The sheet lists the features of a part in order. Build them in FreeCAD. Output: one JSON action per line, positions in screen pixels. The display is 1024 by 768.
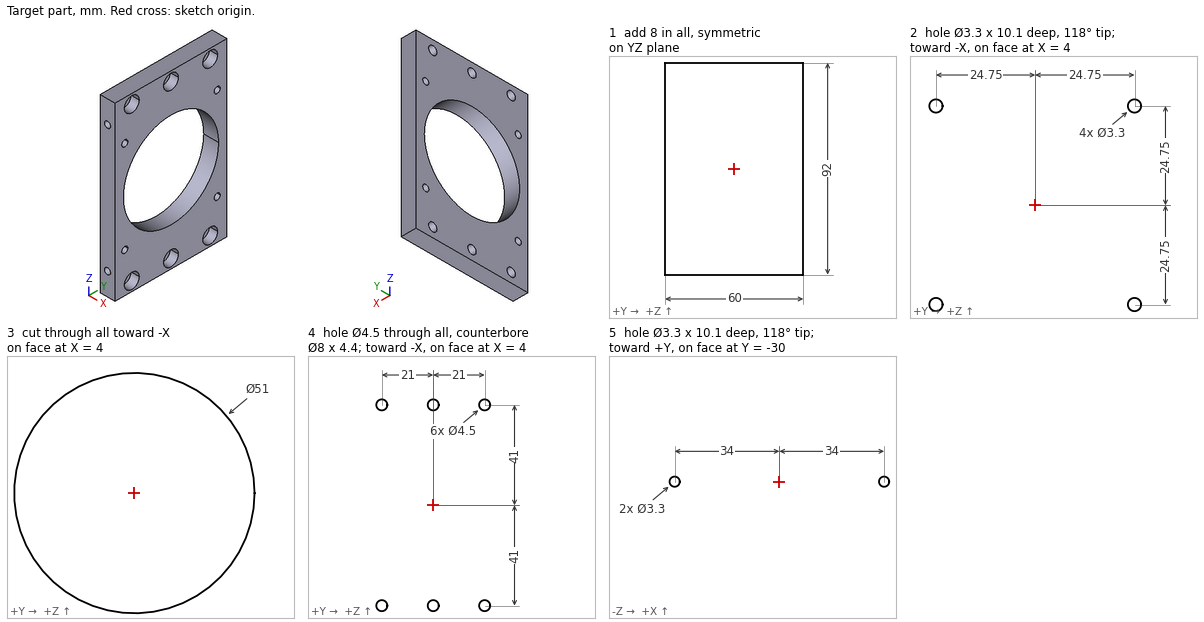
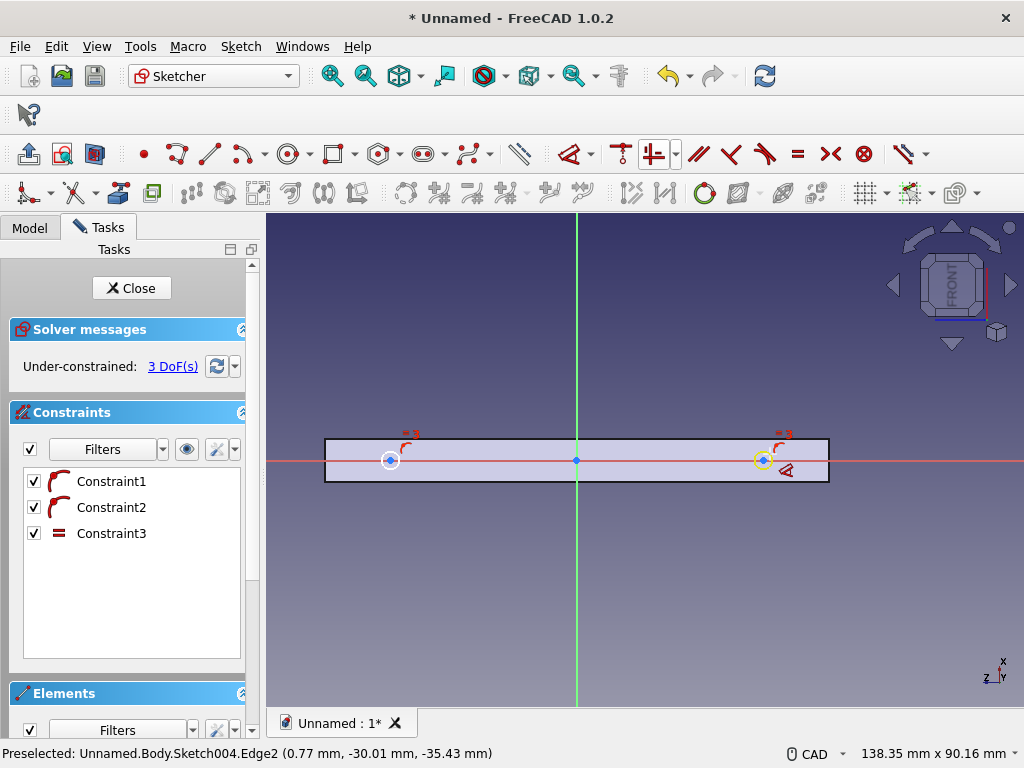
{"action": "scroll", "coordinate": [397, 454], "scroll_direction": "up", "scroll_amount": 4}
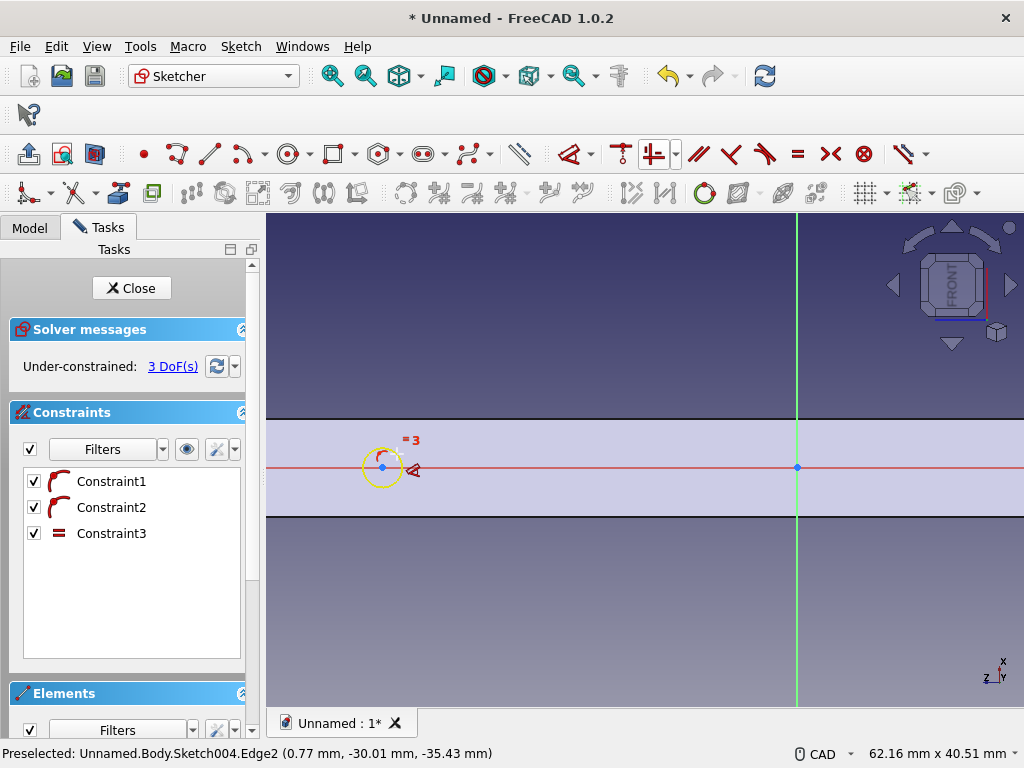
{"action": "left_click", "coordinate": [396, 454]}
{"action": "left_click", "coordinate": [418, 431]}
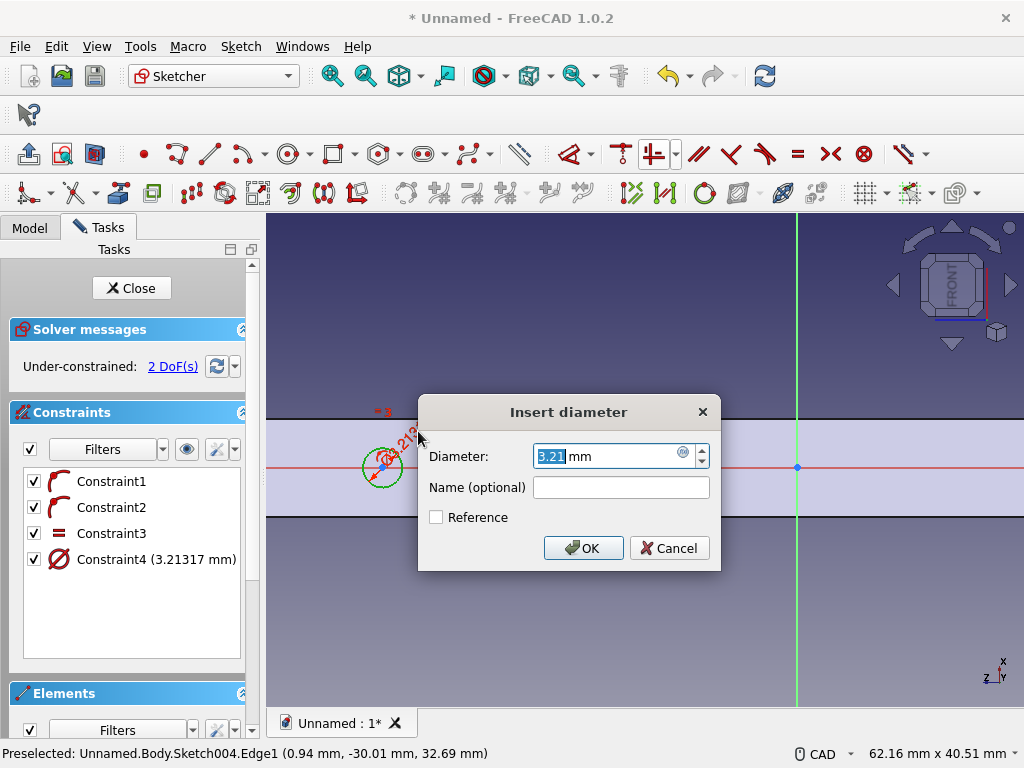
{"action": "type", "text": "3.3"}
{"action": "key", "text": "Return"}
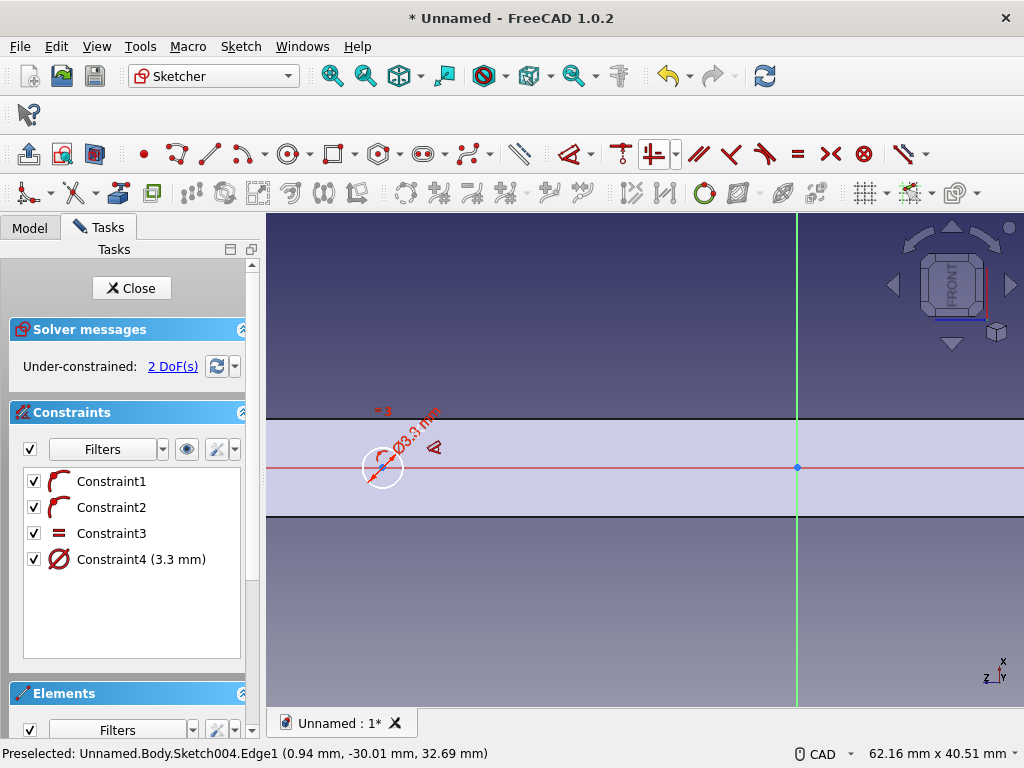
{"action": "left_click", "coordinate": [383, 468]}
{"action": "left_click", "coordinate": [590, 502]}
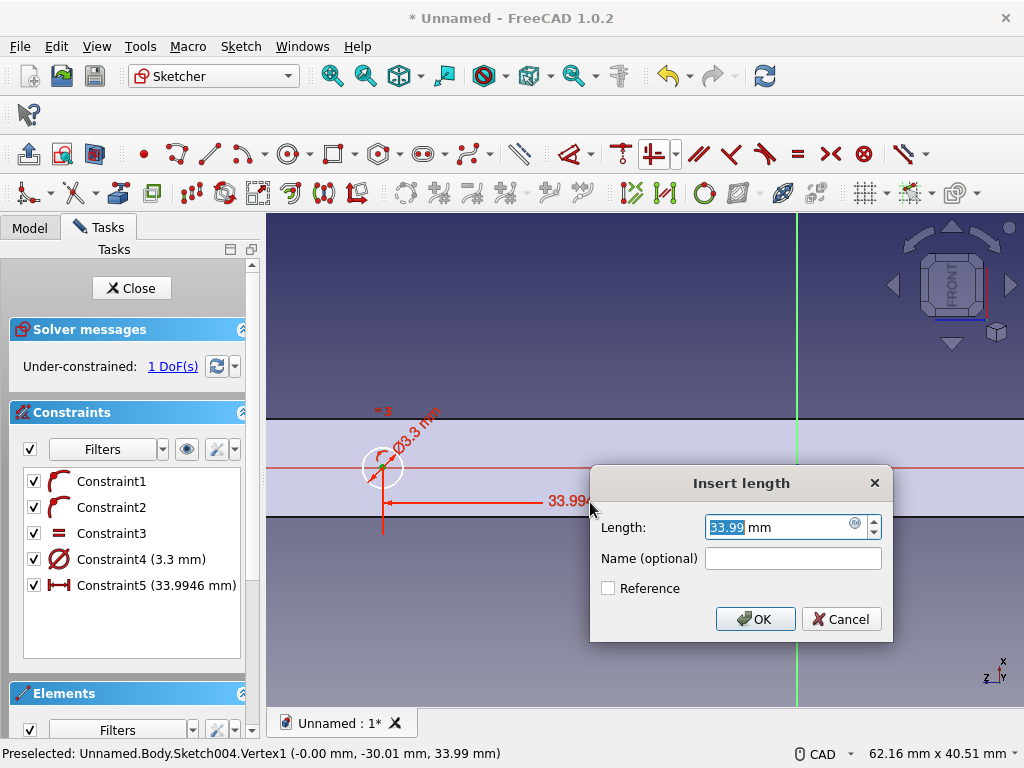
{"action": "type", "text": "34"}
{"action": "key", "text": "Return"}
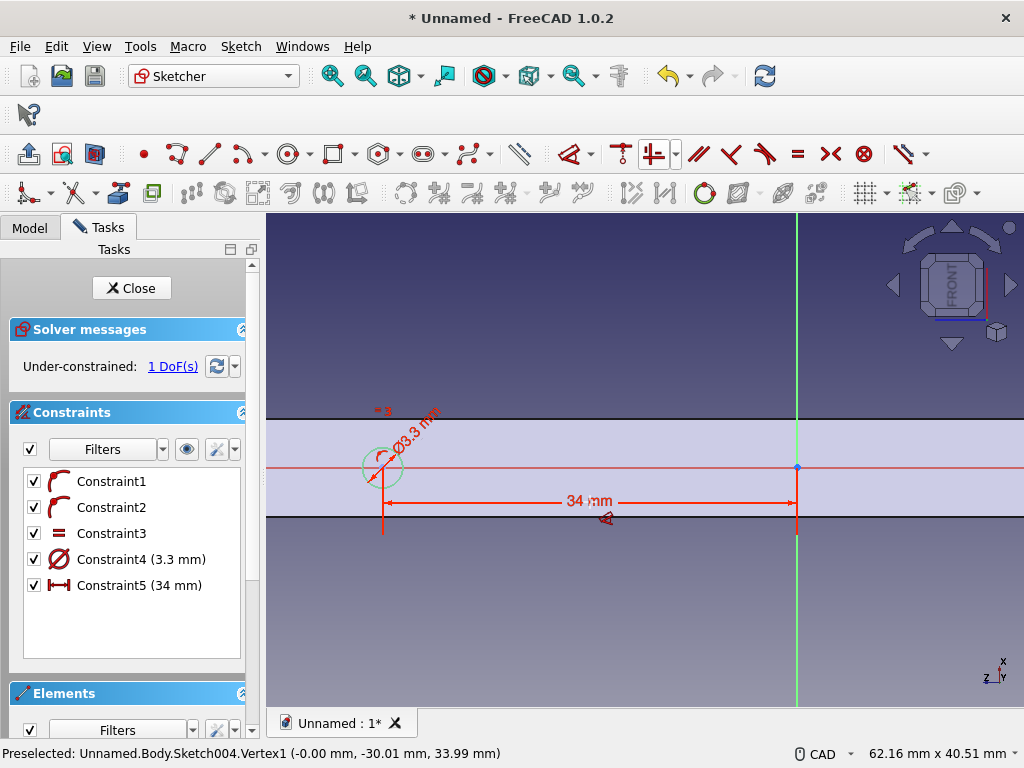
{"action": "scroll", "coordinate": [396, 454], "scroll_direction": "down", "scroll_amount": 4}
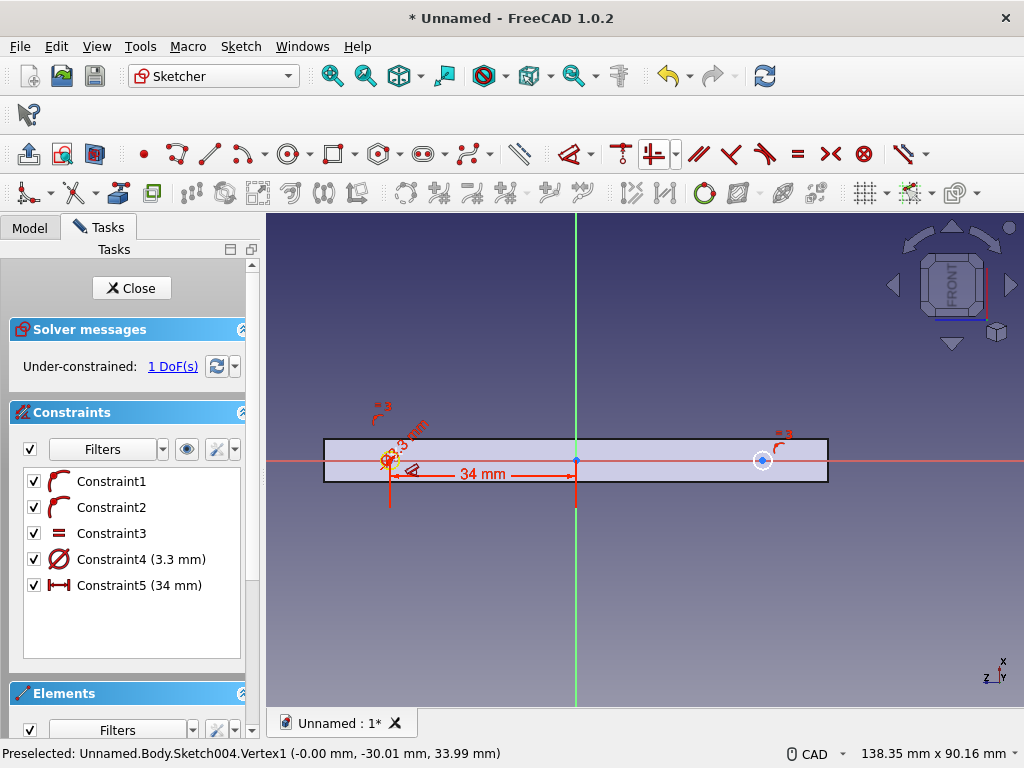
{"action": "left_click", "coordinate": [763, 461]}
{"action": "left_click", "coordinate": [670, 495]}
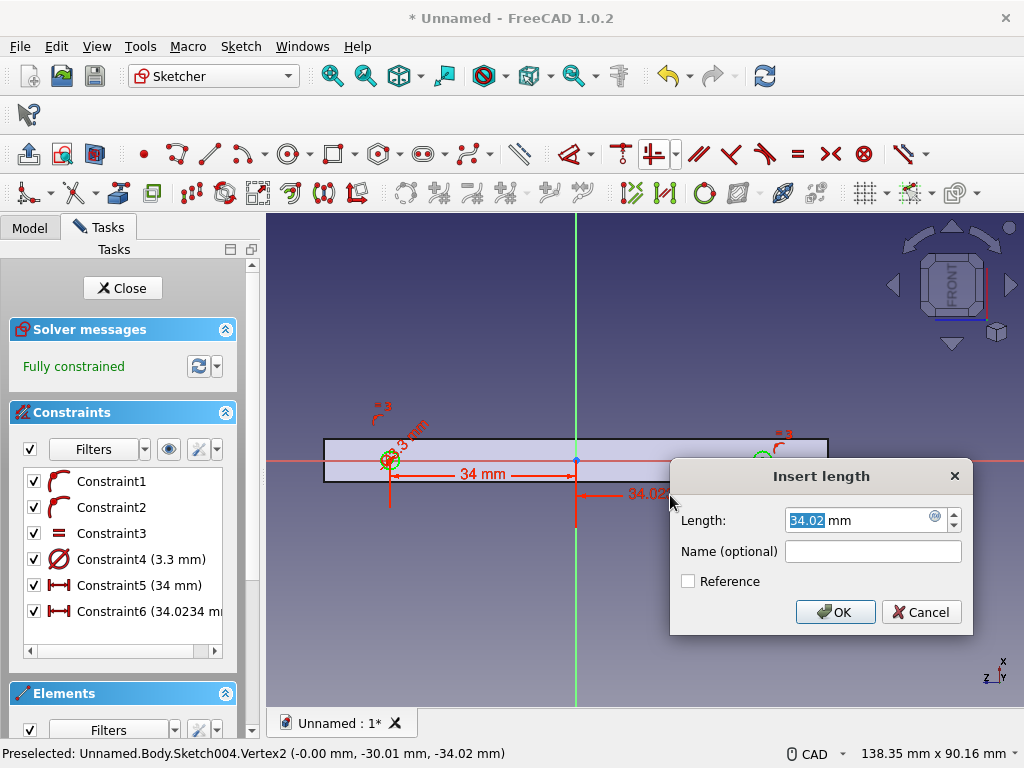
{"action": "type", "text": "34"}
{"action": "key", "text": "Return"}
{"action": "key", "text": "Escape"}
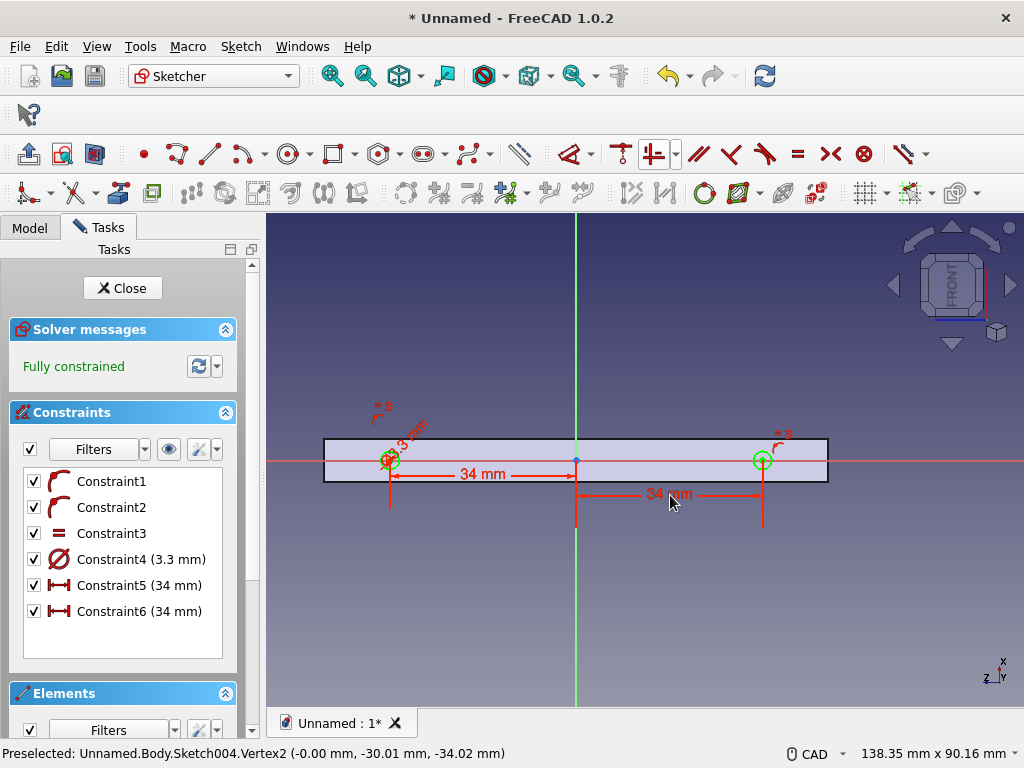
{"action": "left_click", "coordinate": [123, 288]}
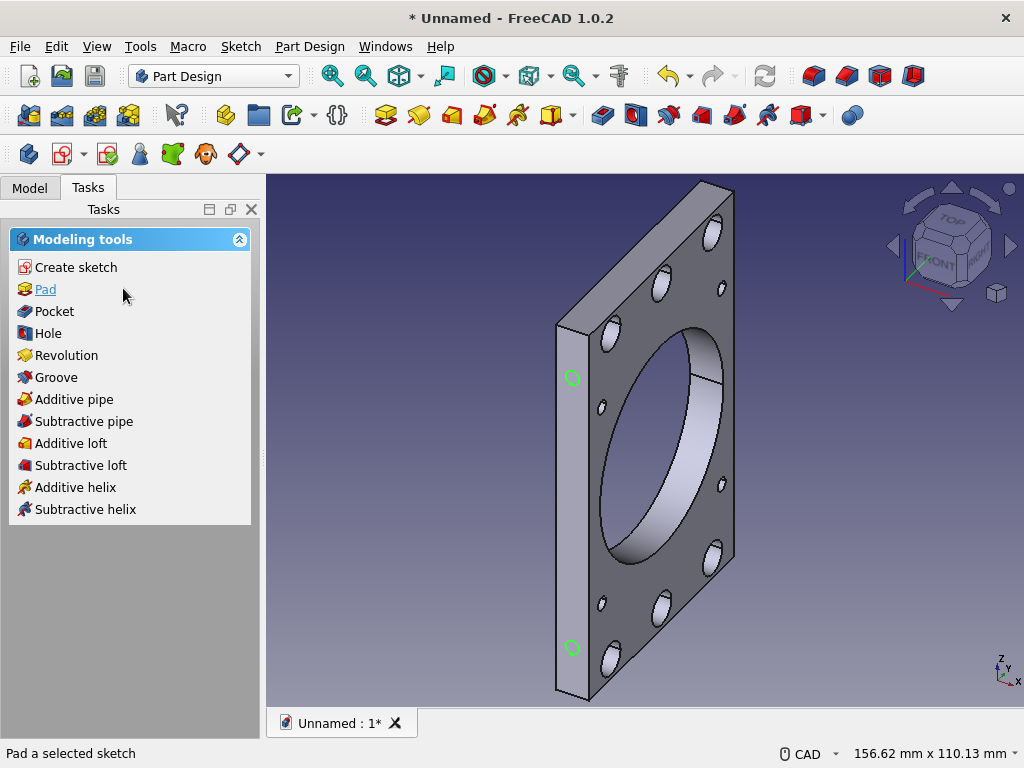
{"action": "left_click", "coordinate": [636, 116]}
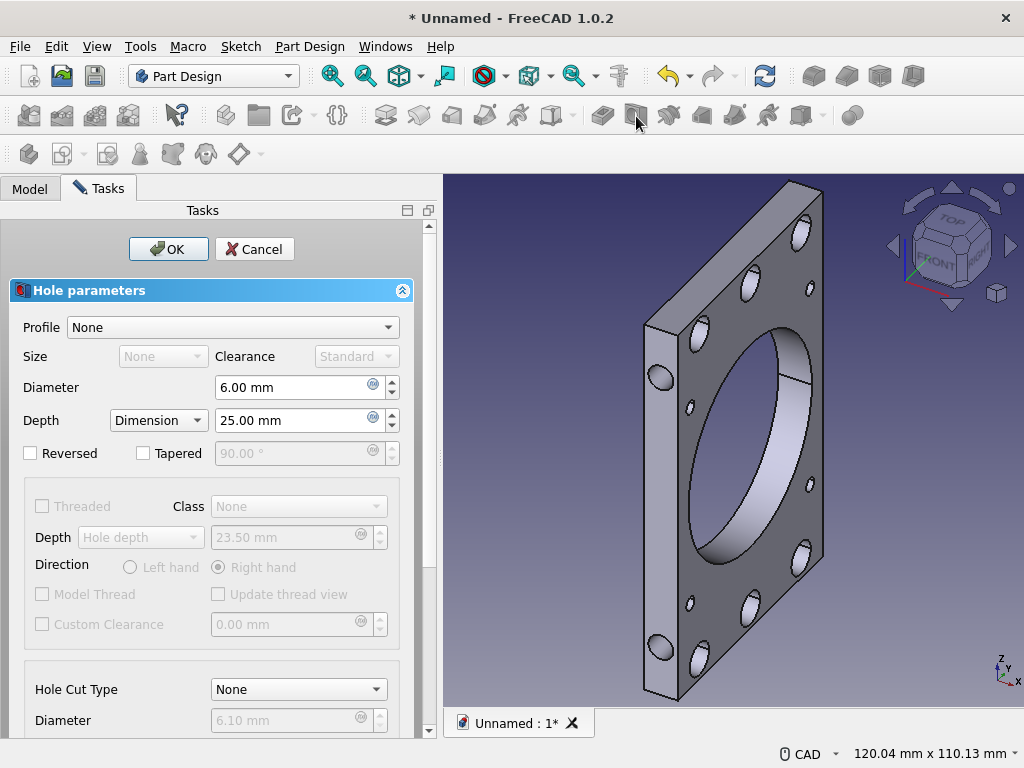
{"action": "triple_click", "coordinate": [300, 388]}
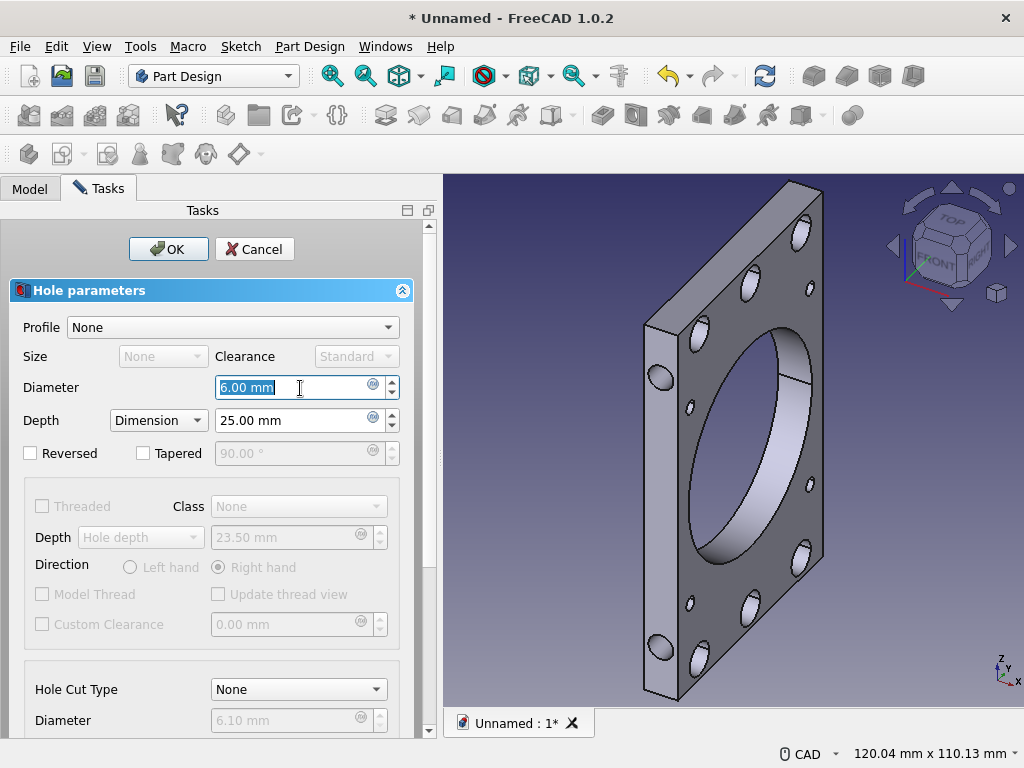
{"action": "type", "text": "3.3"}
{"action": "key", "text": "Tab"}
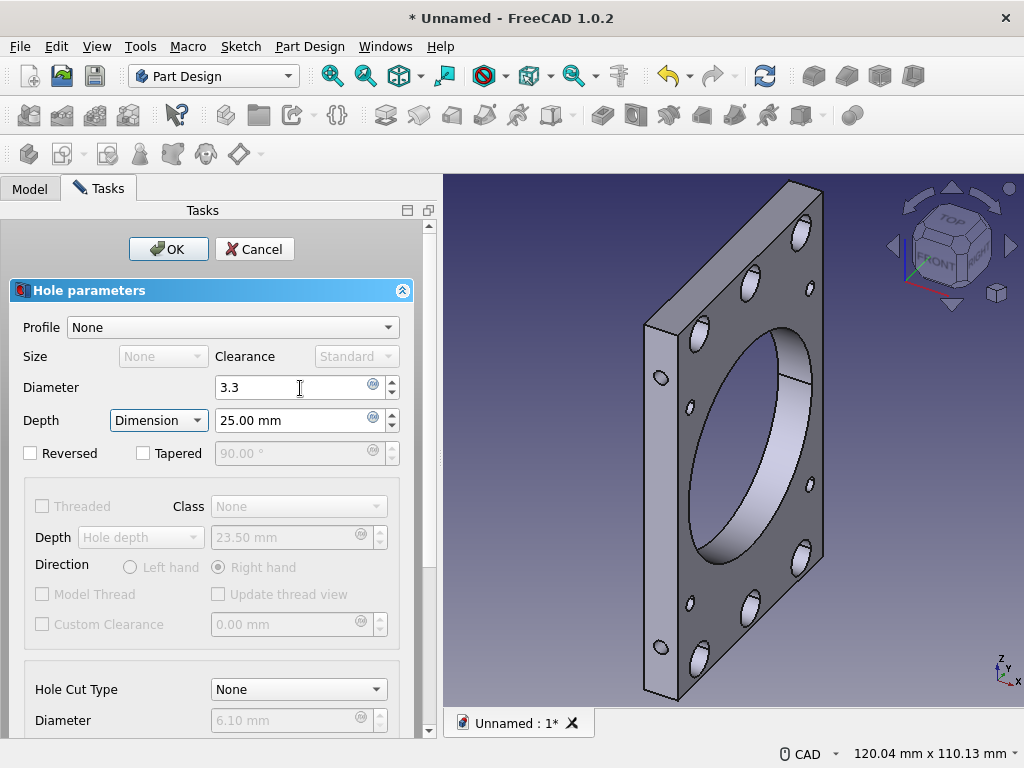
{"action": "triple_click", "coordinate": [300, 420]}